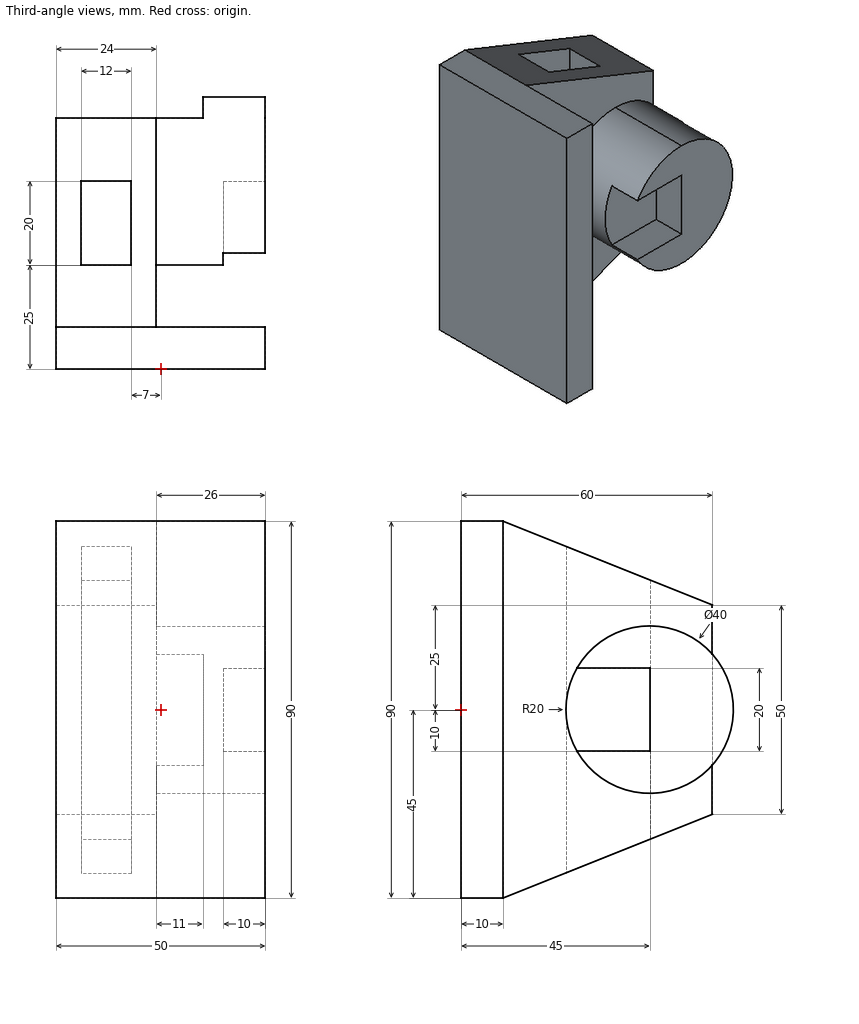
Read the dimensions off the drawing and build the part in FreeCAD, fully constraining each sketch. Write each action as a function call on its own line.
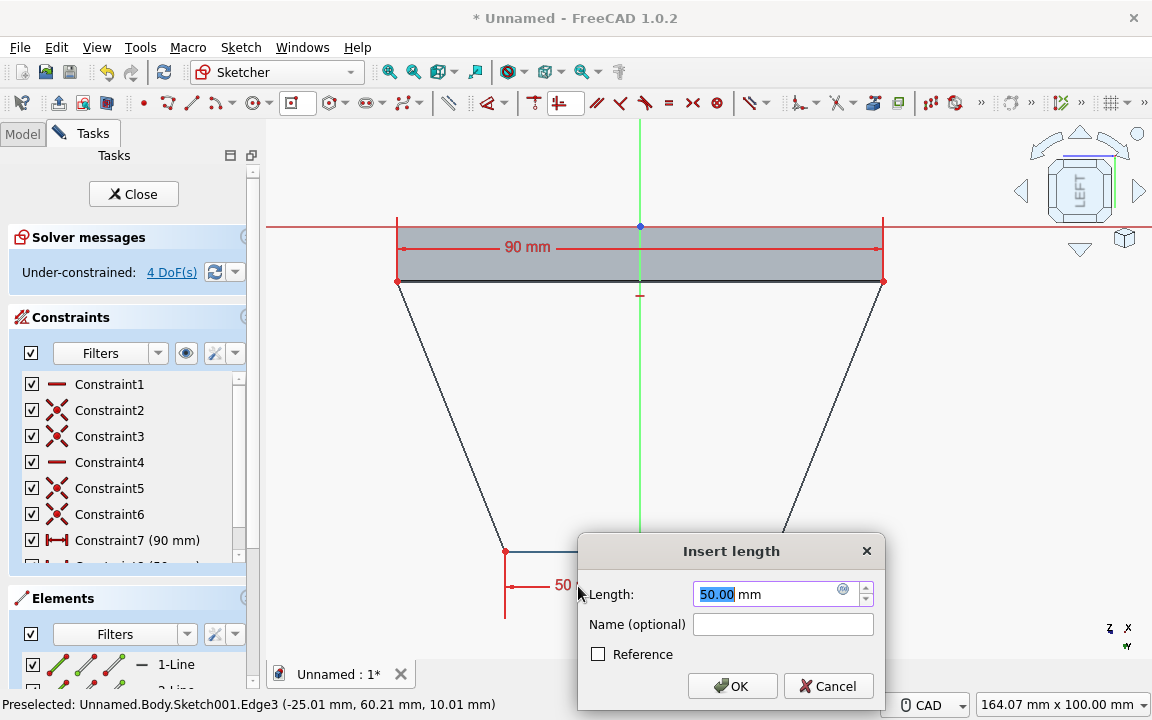
text(50)
key(Return)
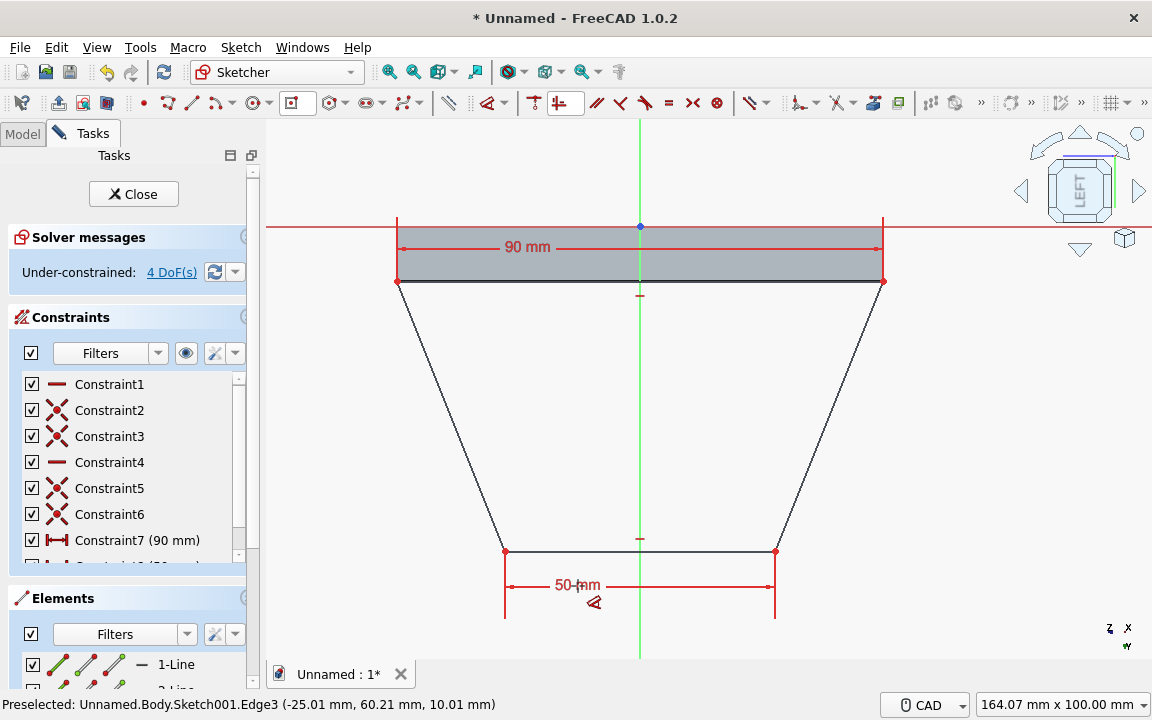
click(883, 282)
click(762, 193)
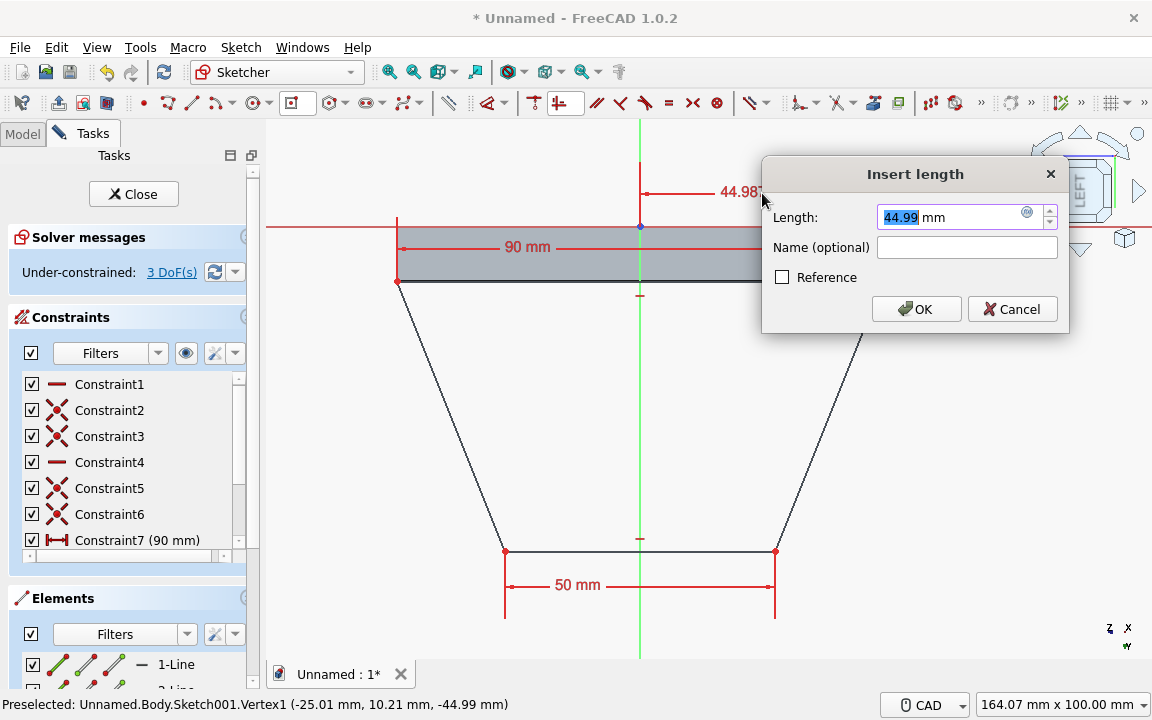
text(45)
key(Return)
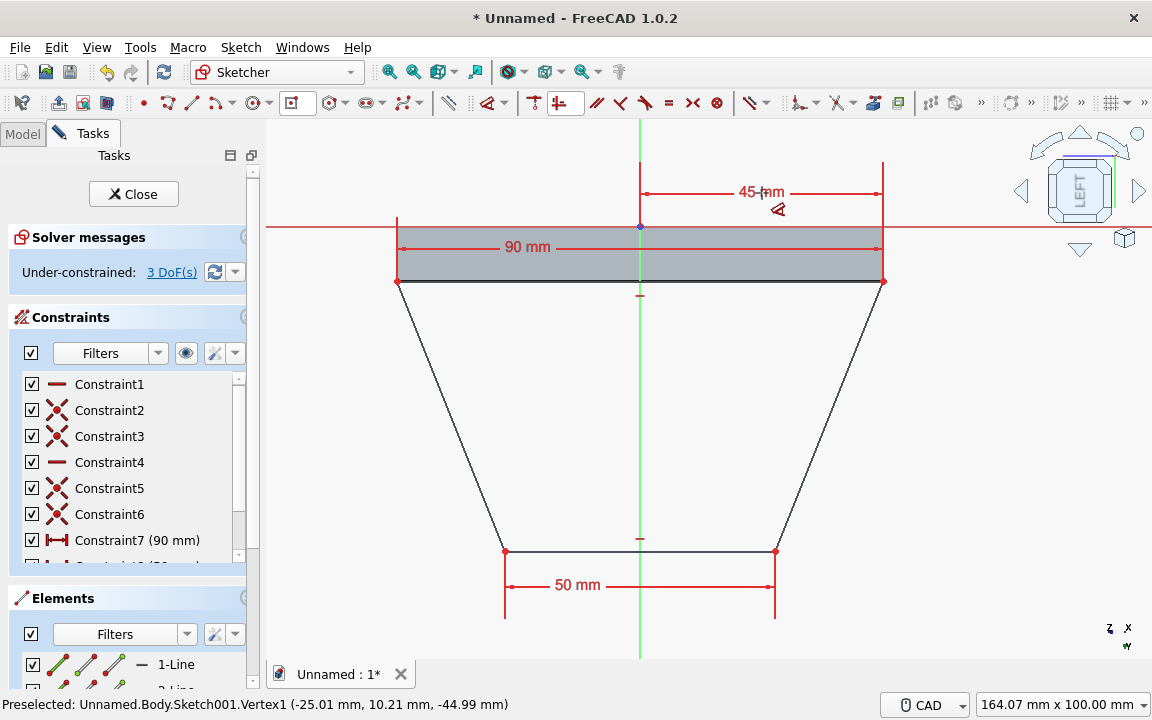
click(883, 282)
click(917, 254)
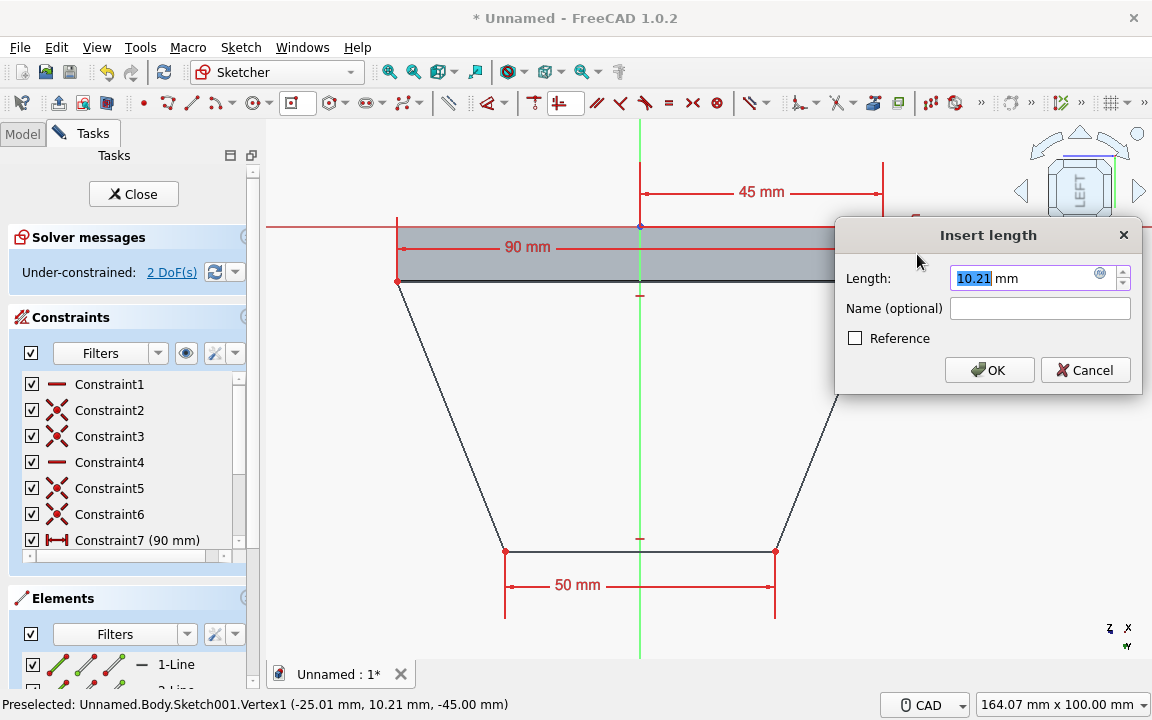
text(10)
key(Return)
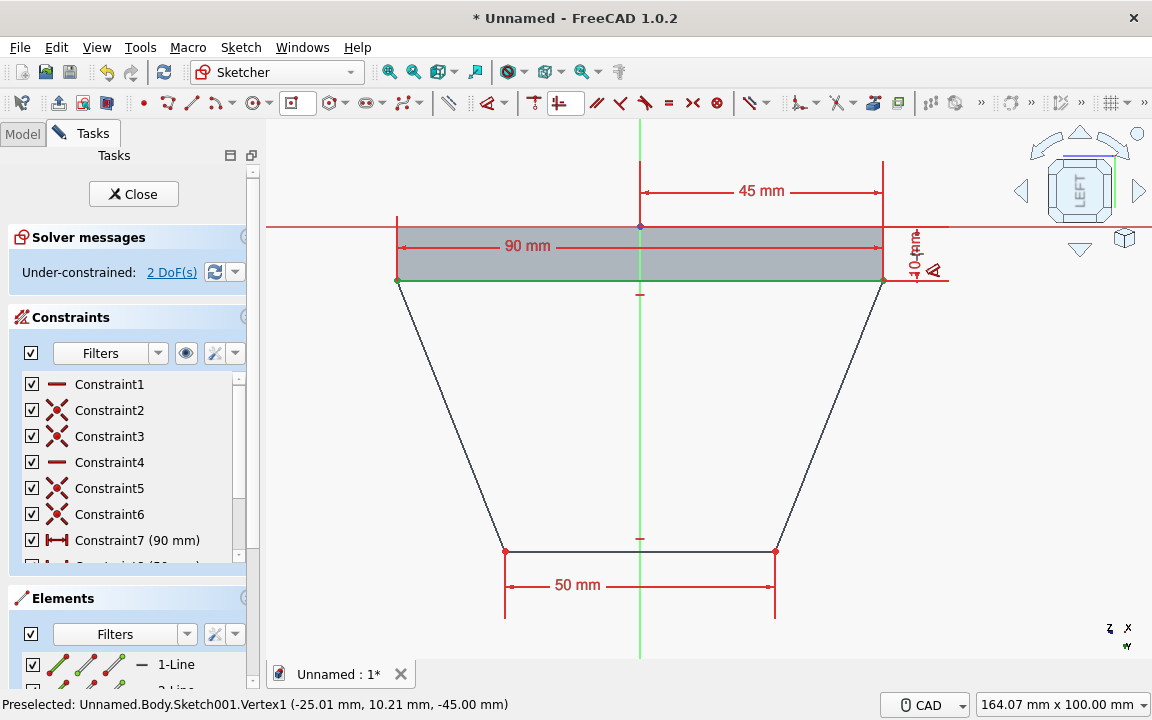
click(505, 552)
click(573, 193)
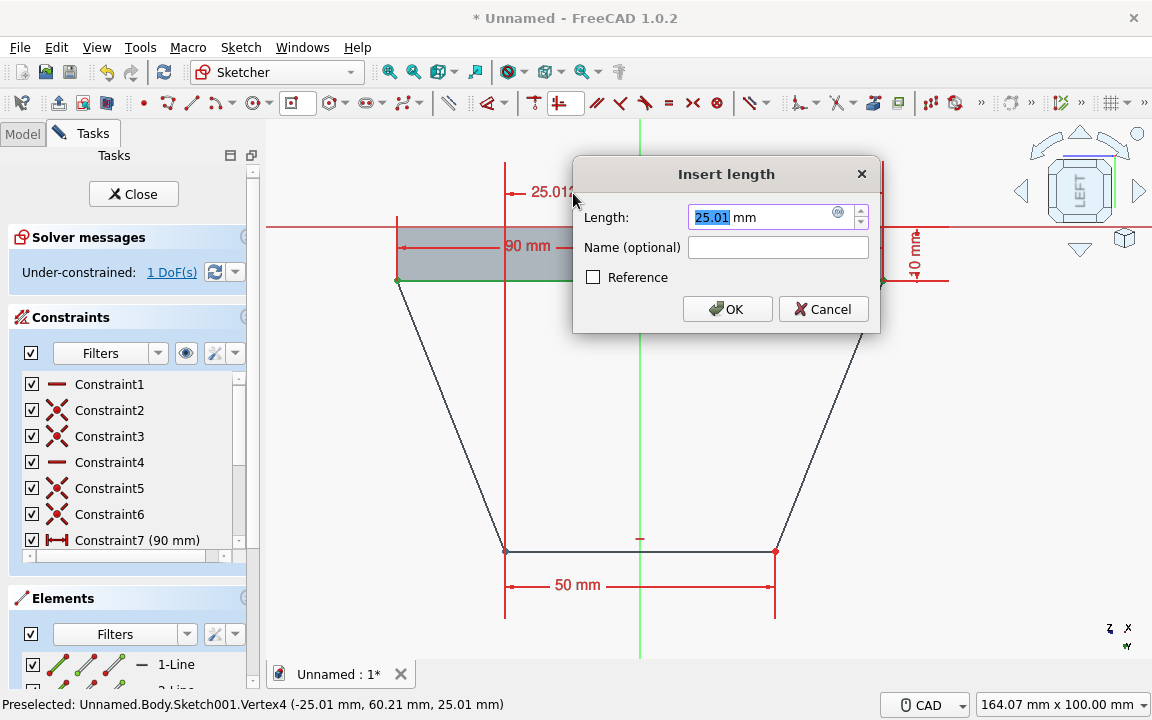
text(25)
key(Return)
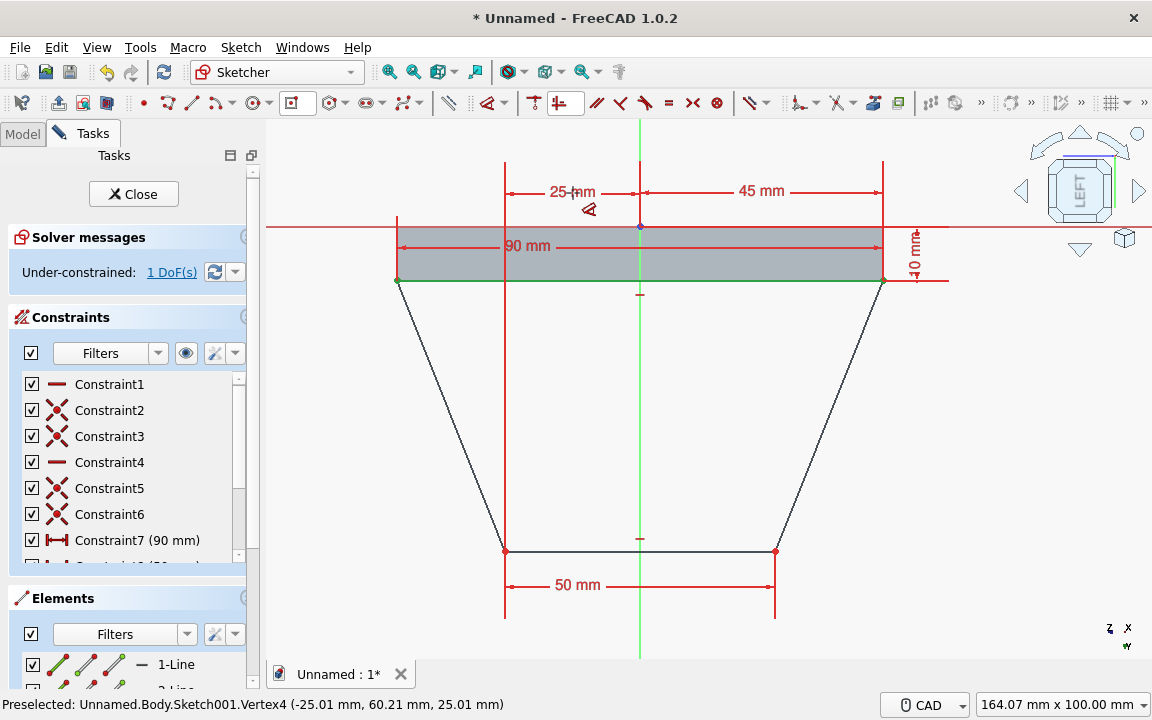
click(505, 552)
click(471, 389)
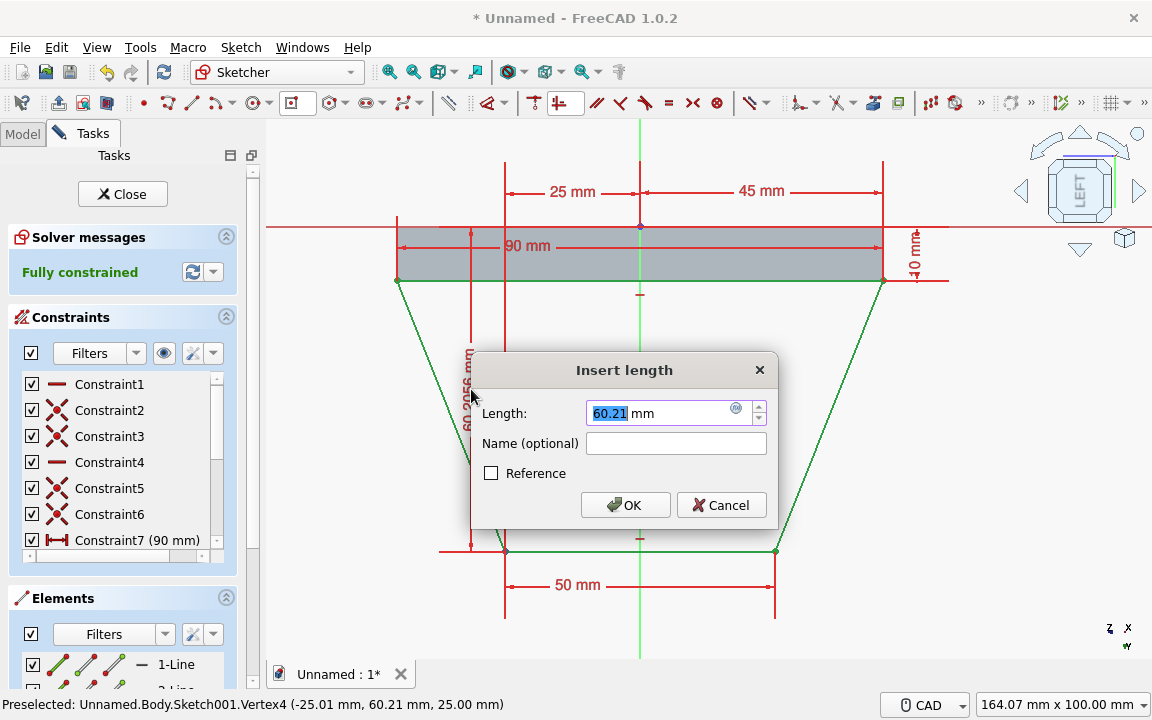
text(60)
key(Return)
key(Escape)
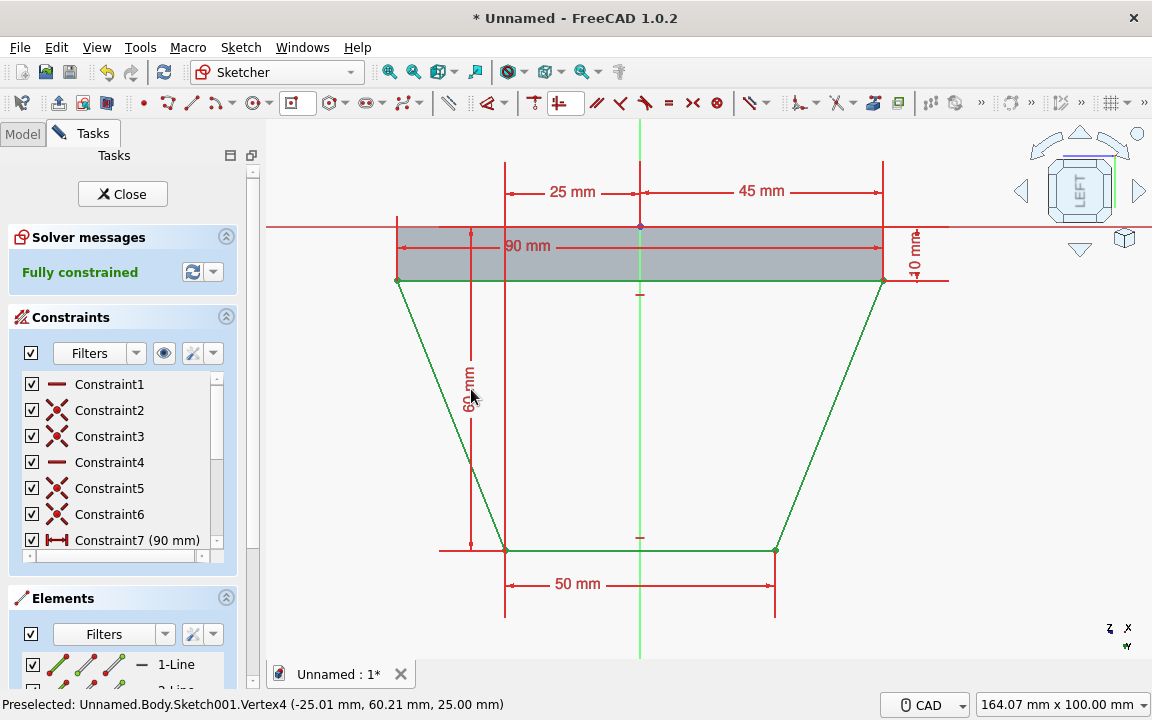
click(123, 194)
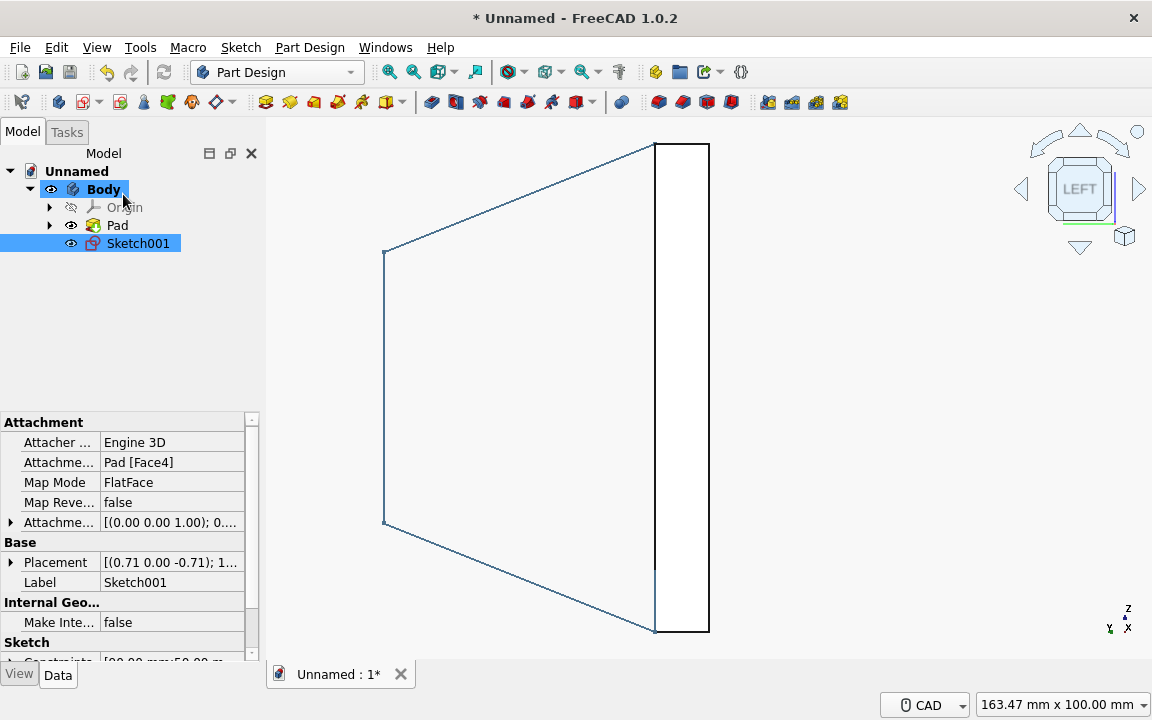
click(266, 102)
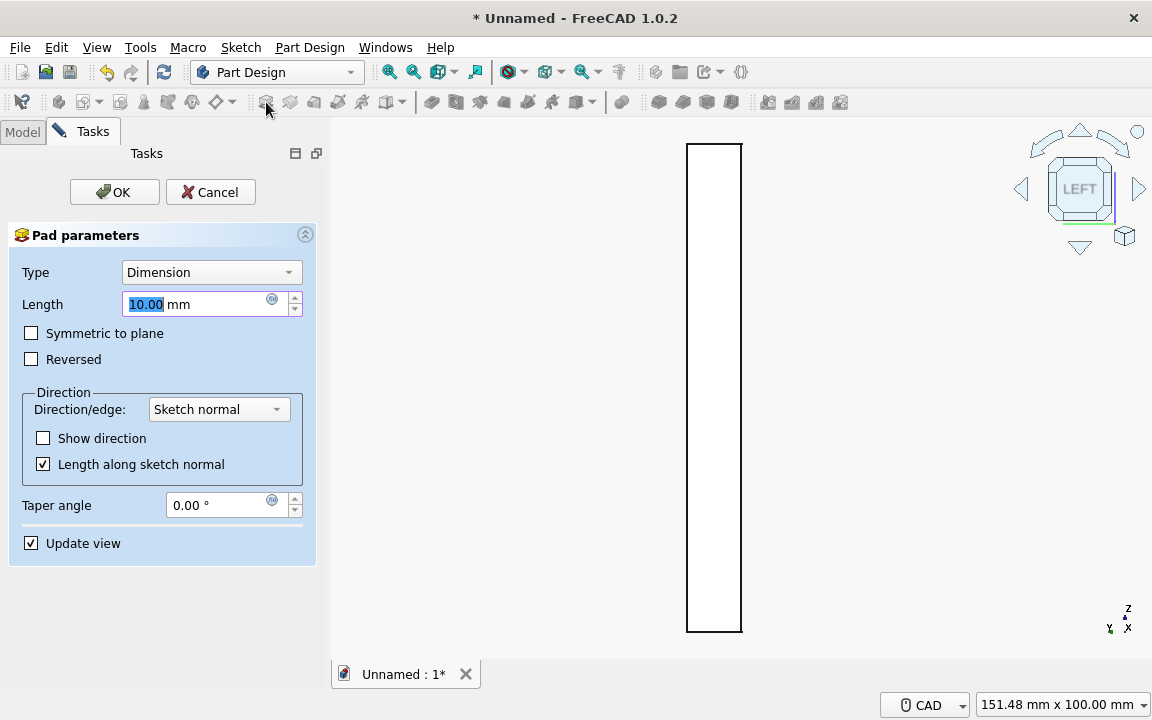
text(24)
key(Tab)